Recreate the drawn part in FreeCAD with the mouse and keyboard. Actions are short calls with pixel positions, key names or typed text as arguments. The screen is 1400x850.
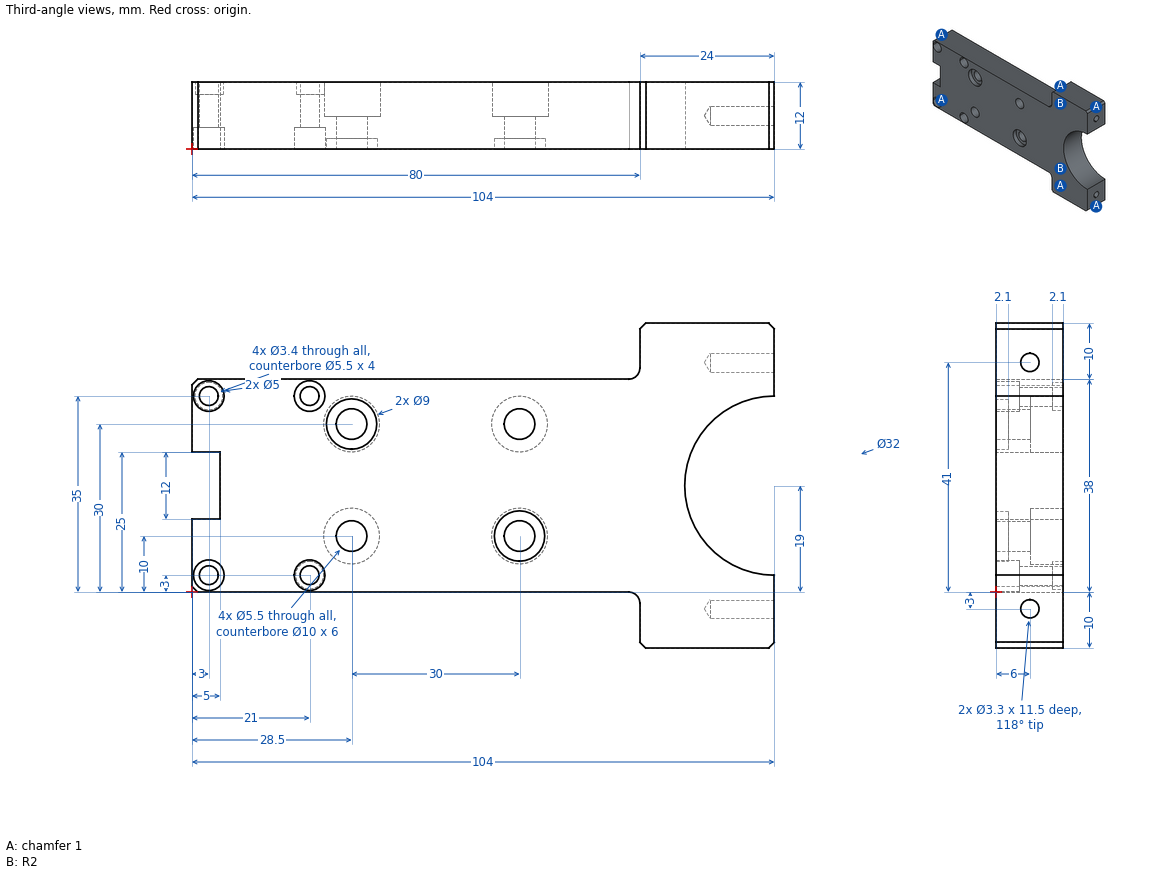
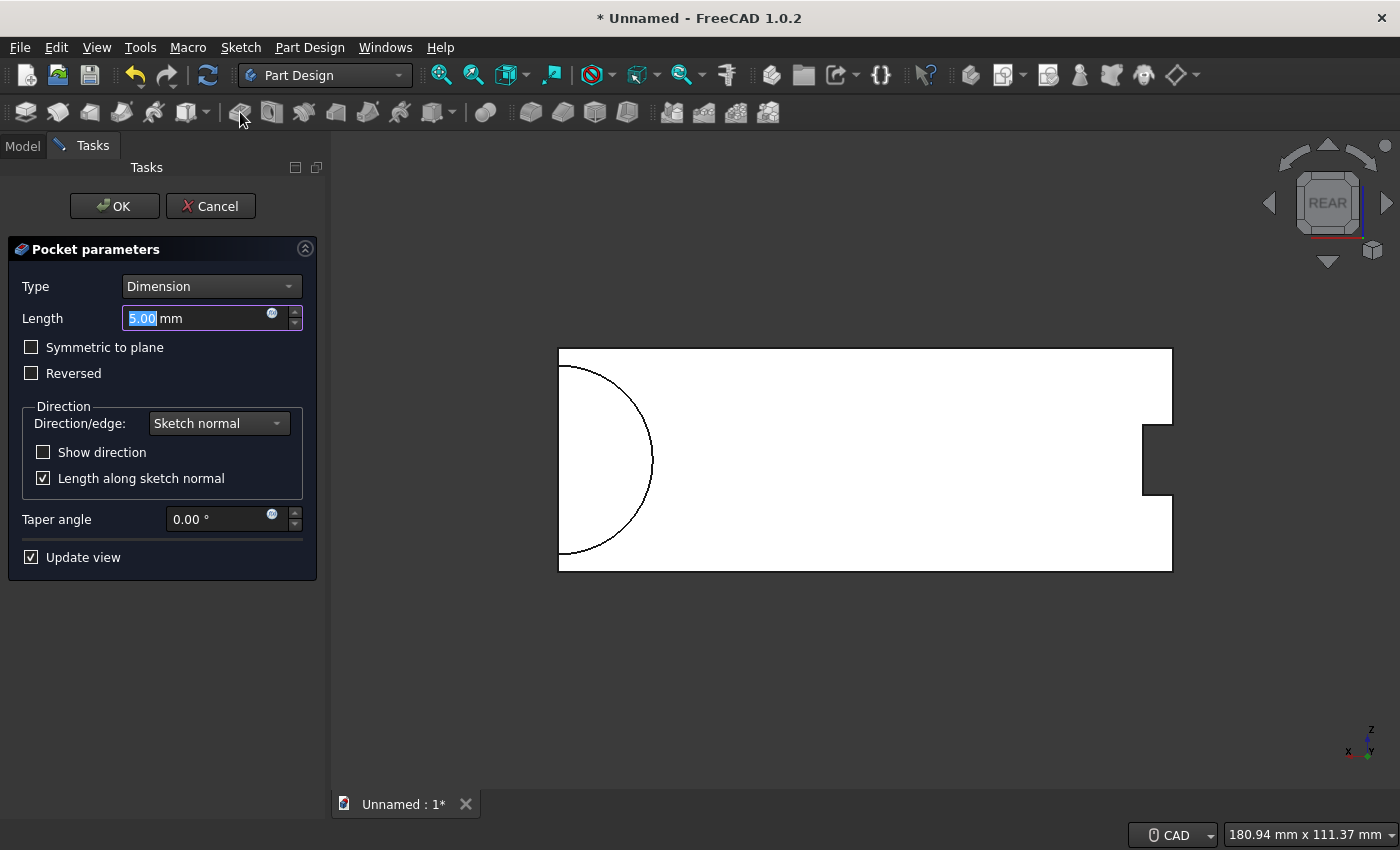
click(212, 286)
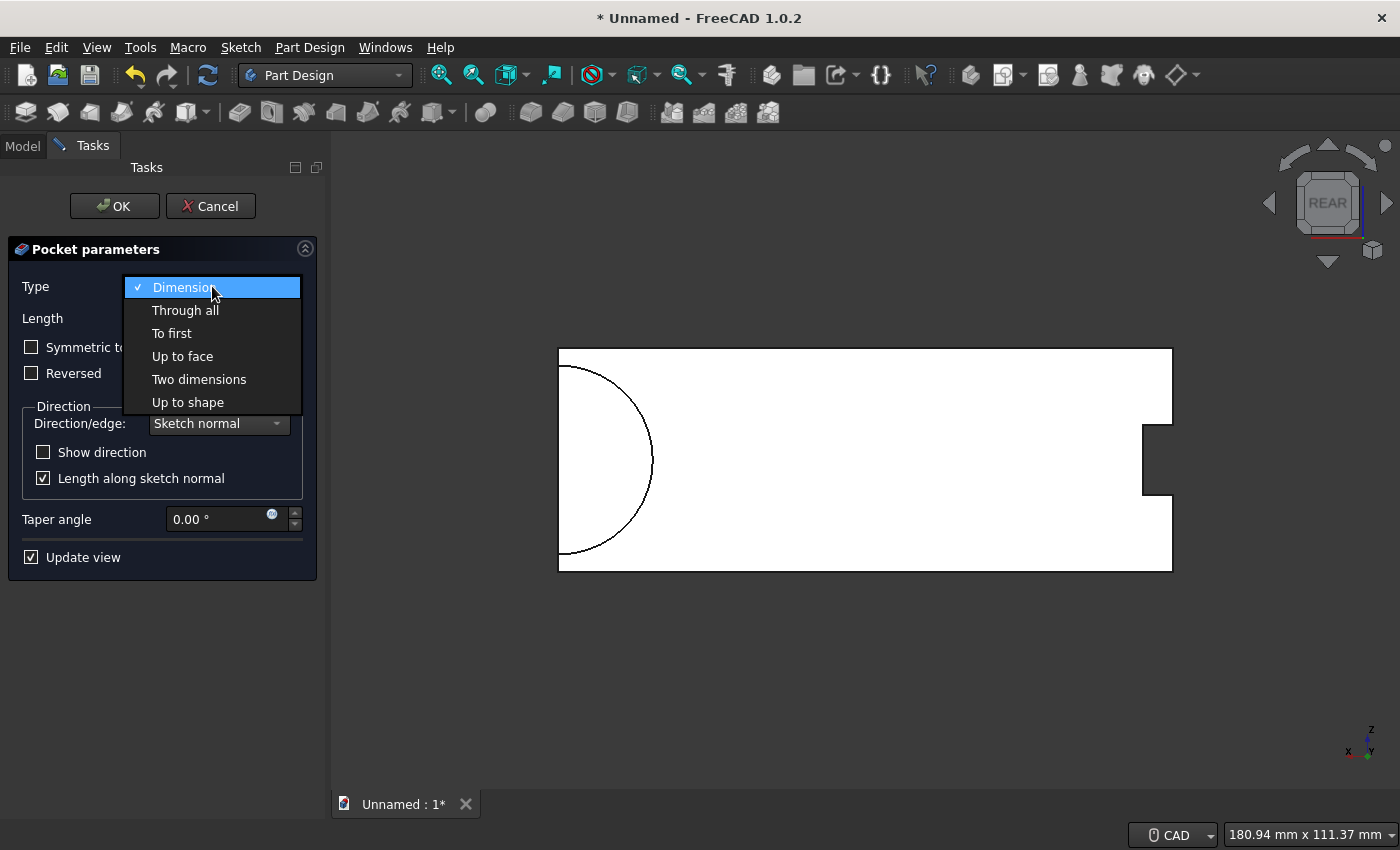
click(212, 310)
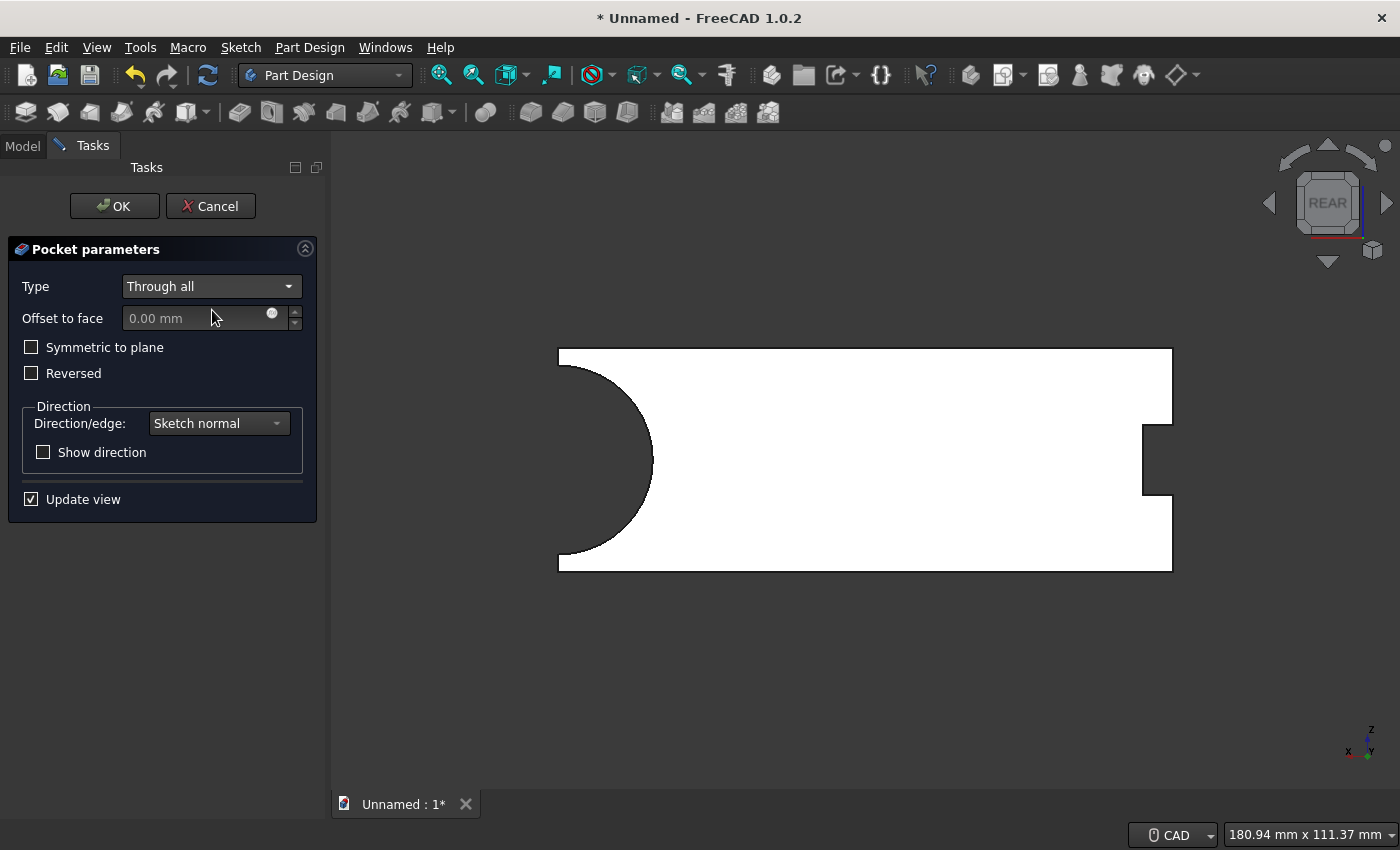
click(115, 206)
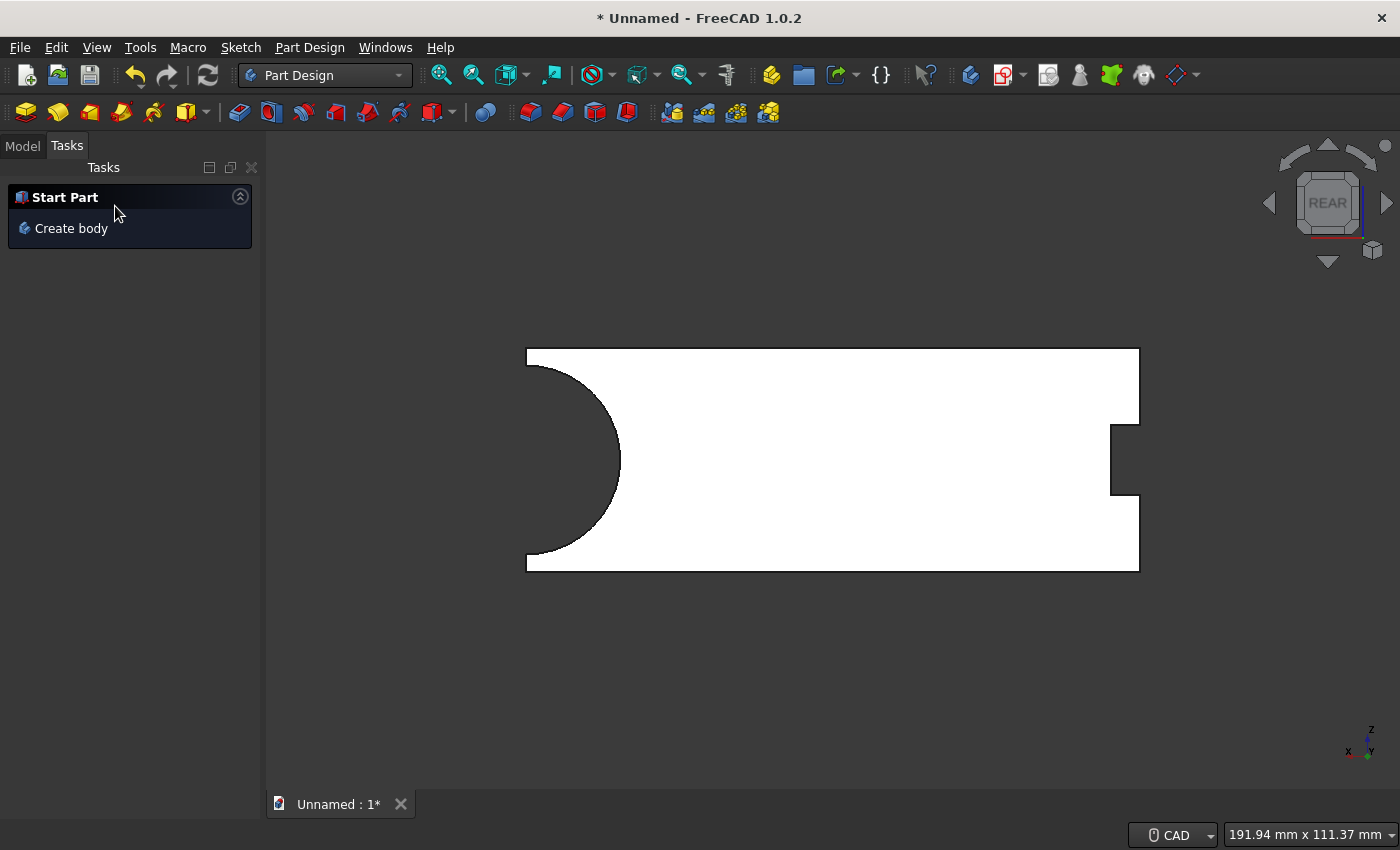
key(5)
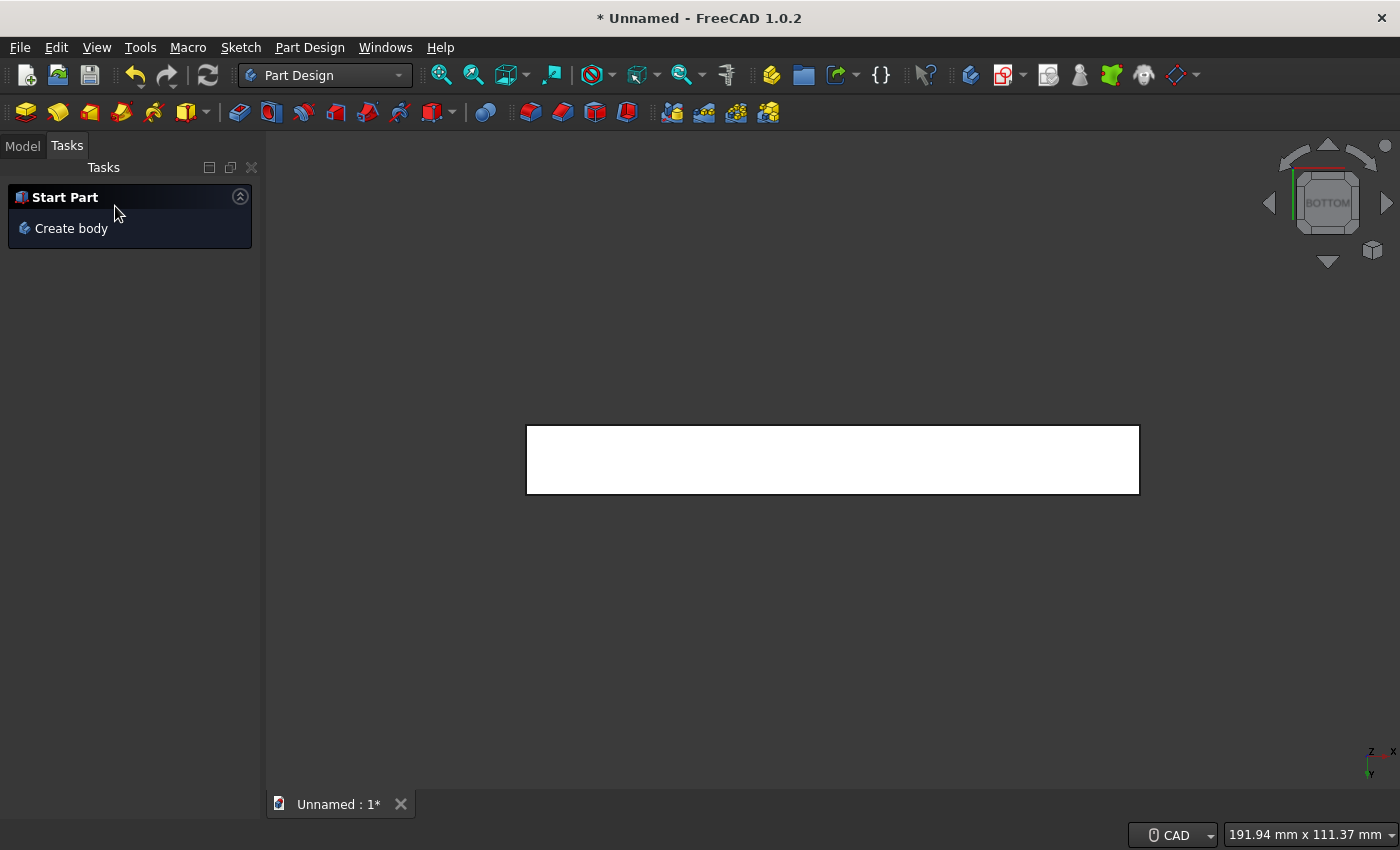
click(1096, 459)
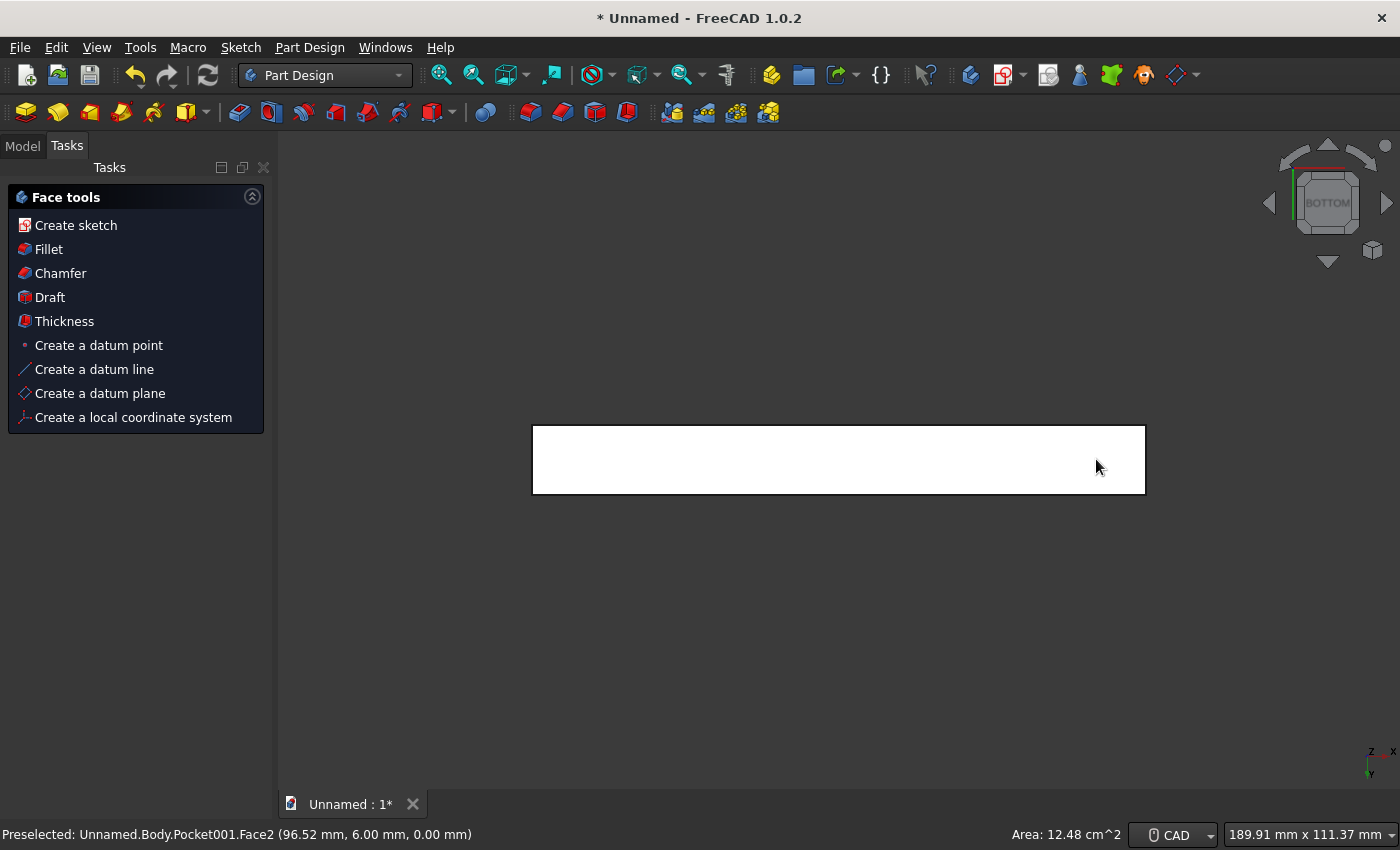
click(1004, 76)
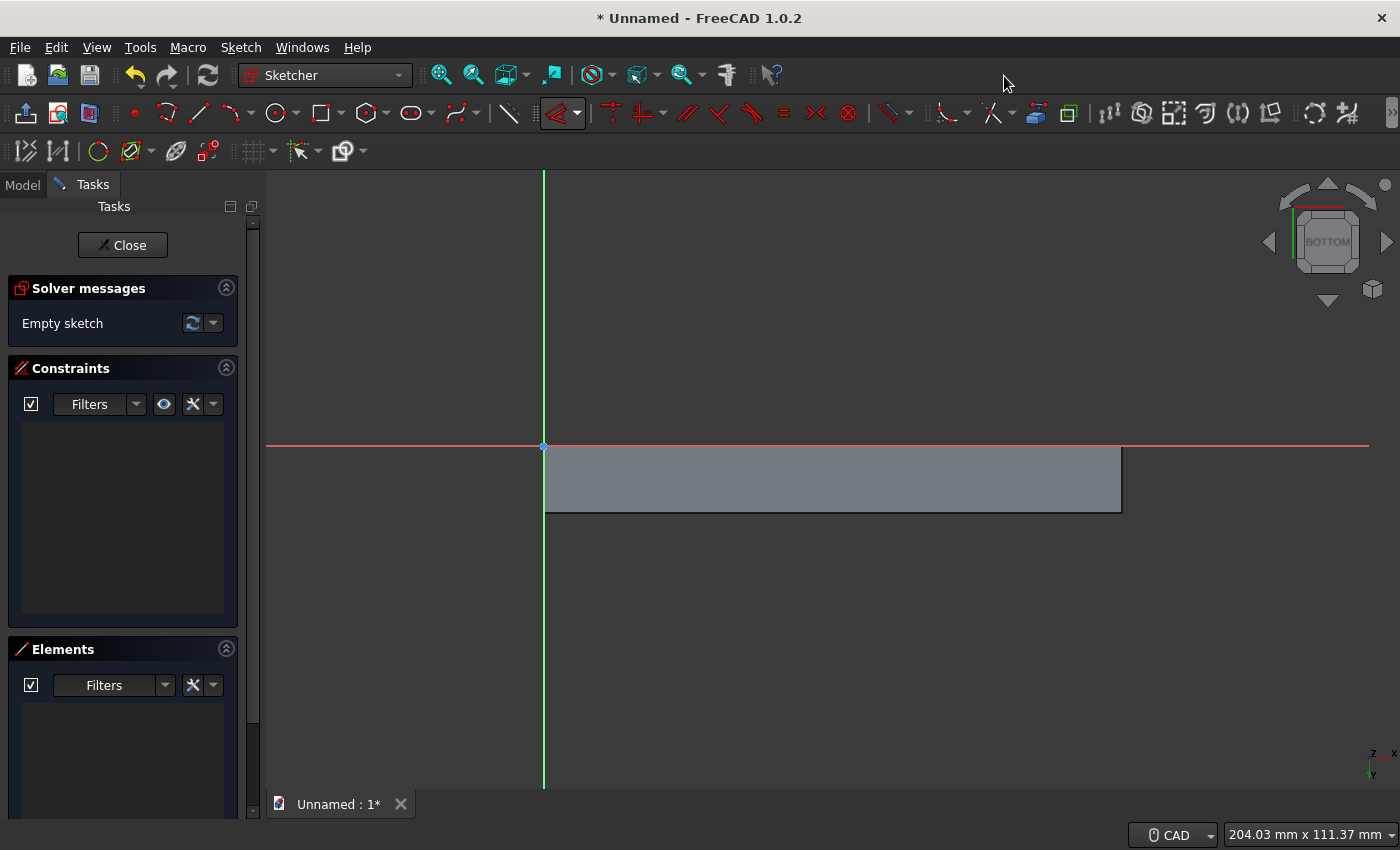
scroll(1129, 480, up, 8)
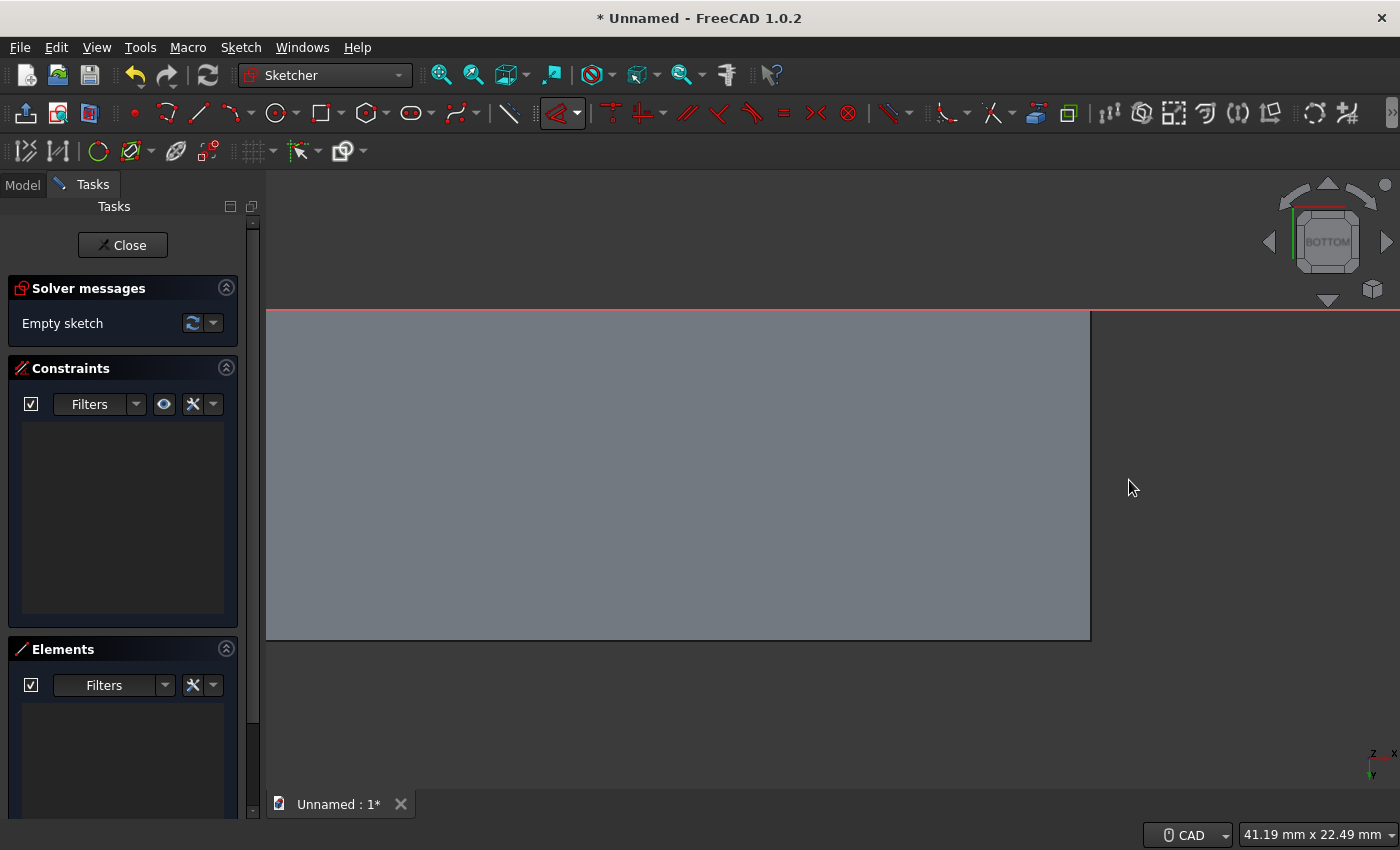
click(322, 114)